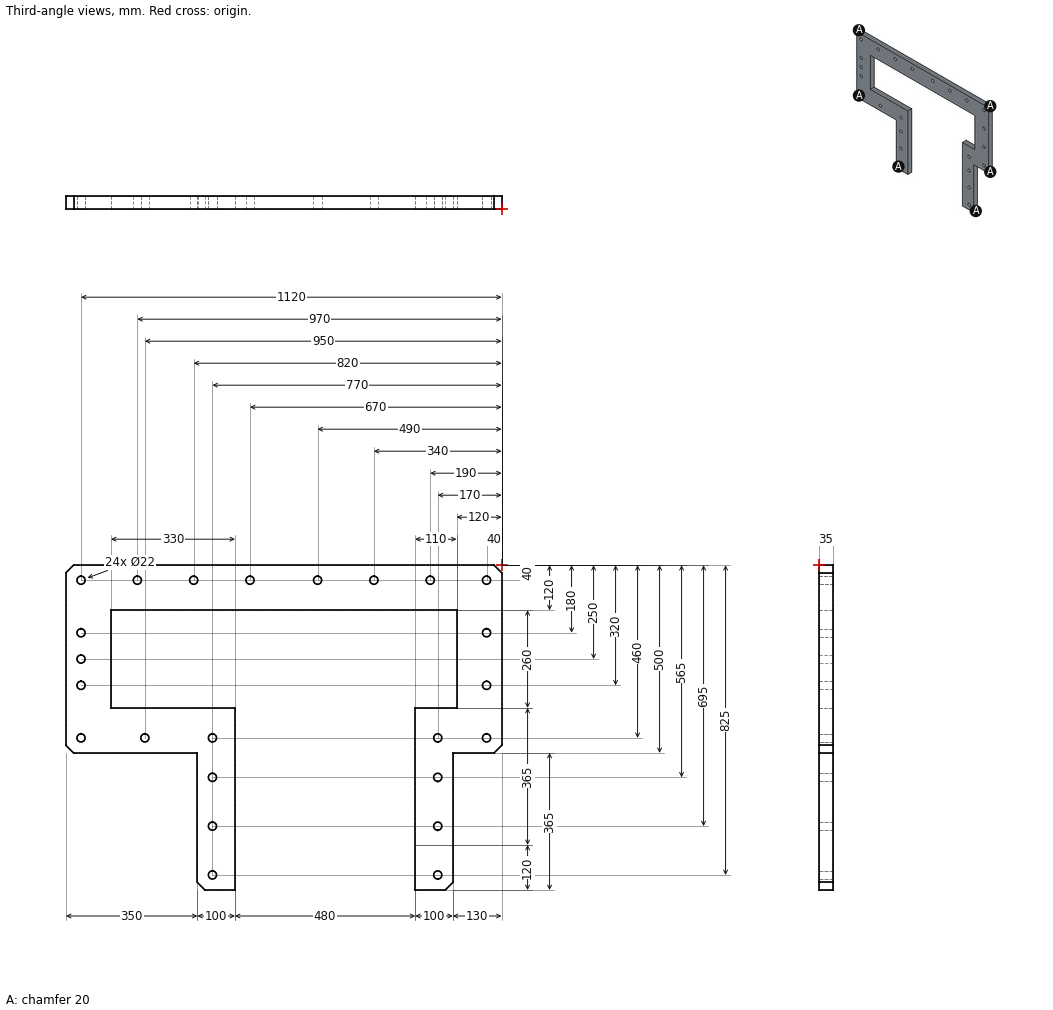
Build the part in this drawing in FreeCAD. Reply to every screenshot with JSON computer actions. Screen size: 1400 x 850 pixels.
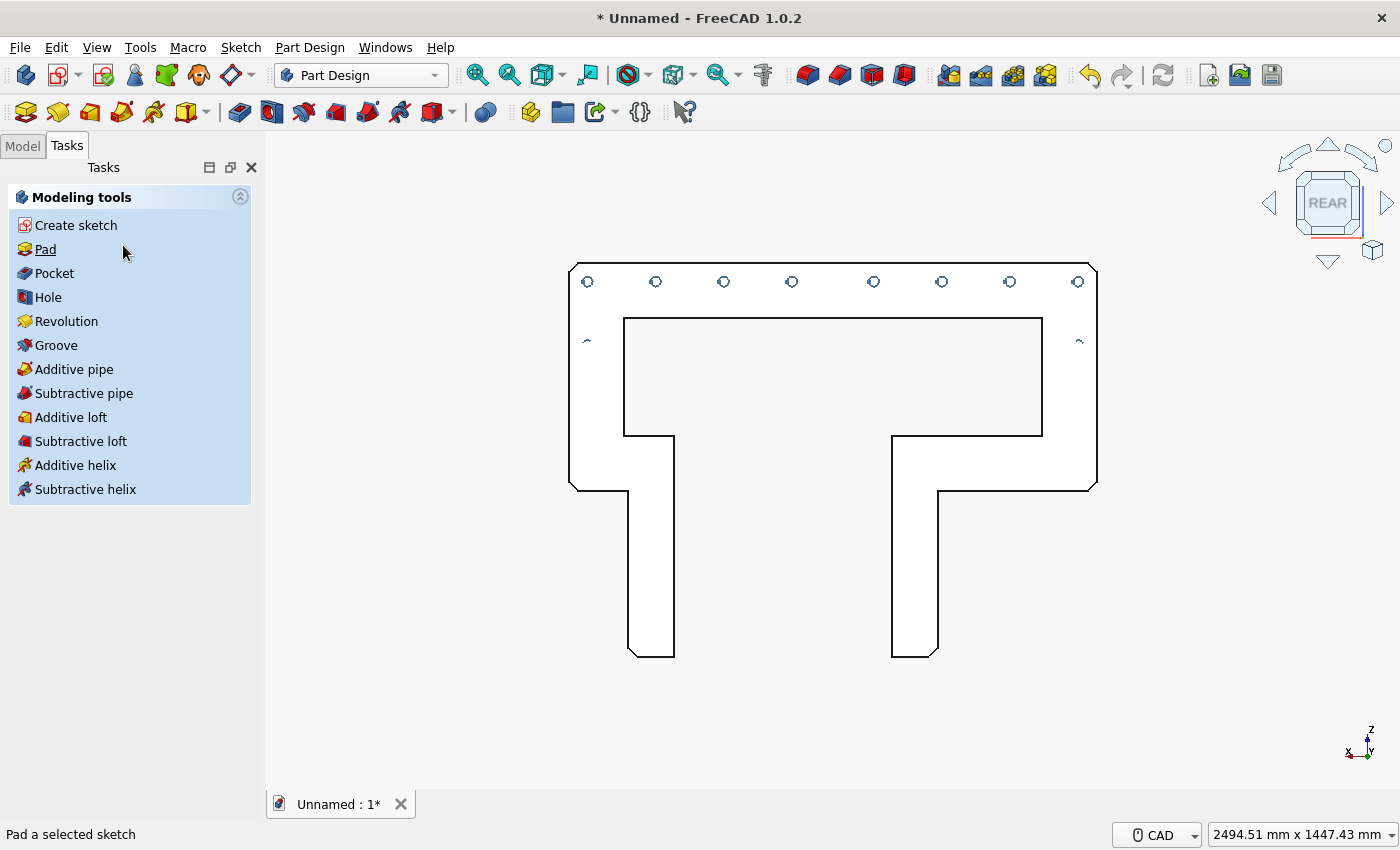
{"action": "left_click", "coordinate": [240, 112]}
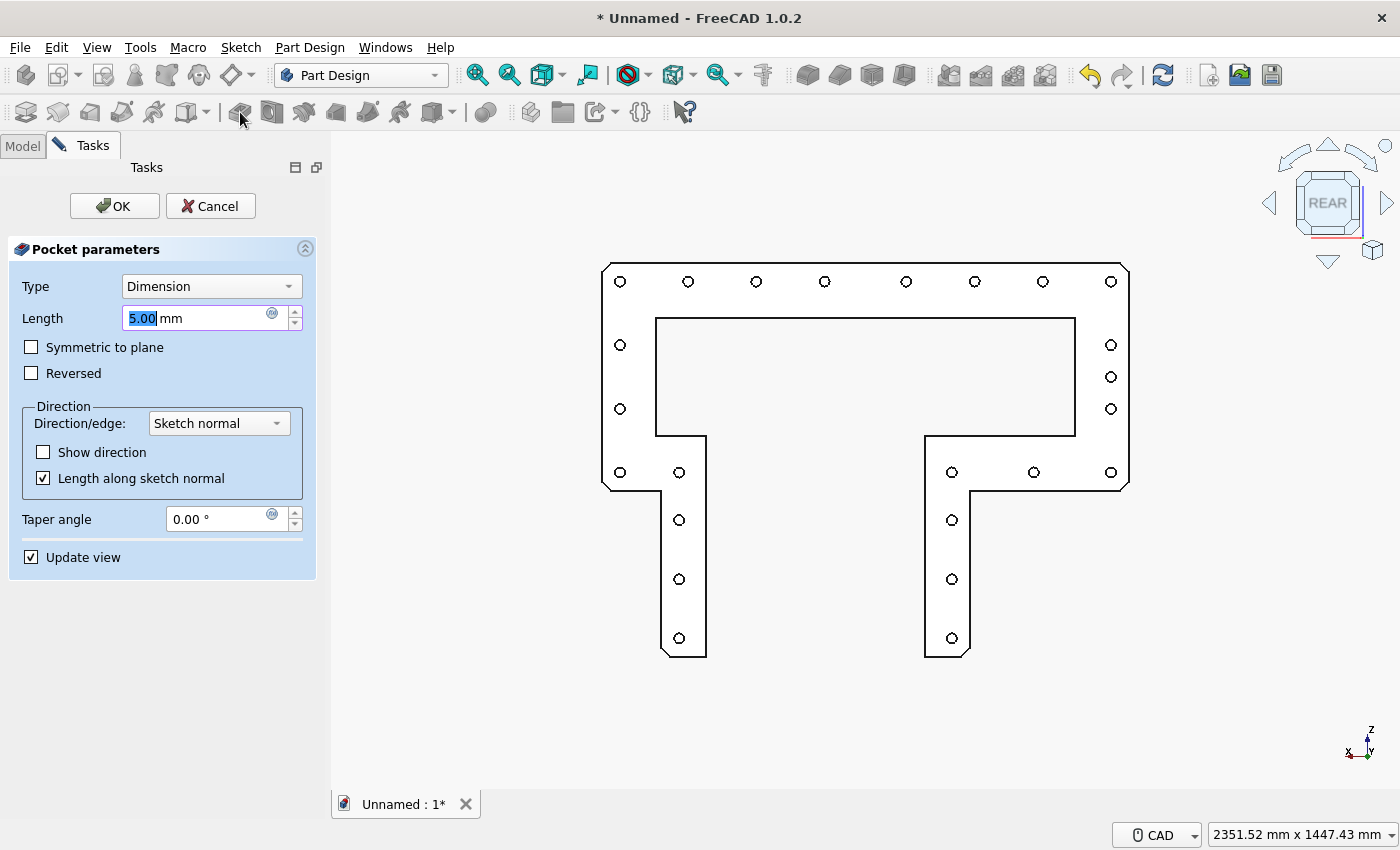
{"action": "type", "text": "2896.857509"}
{"action": "key", "text": "Tab"}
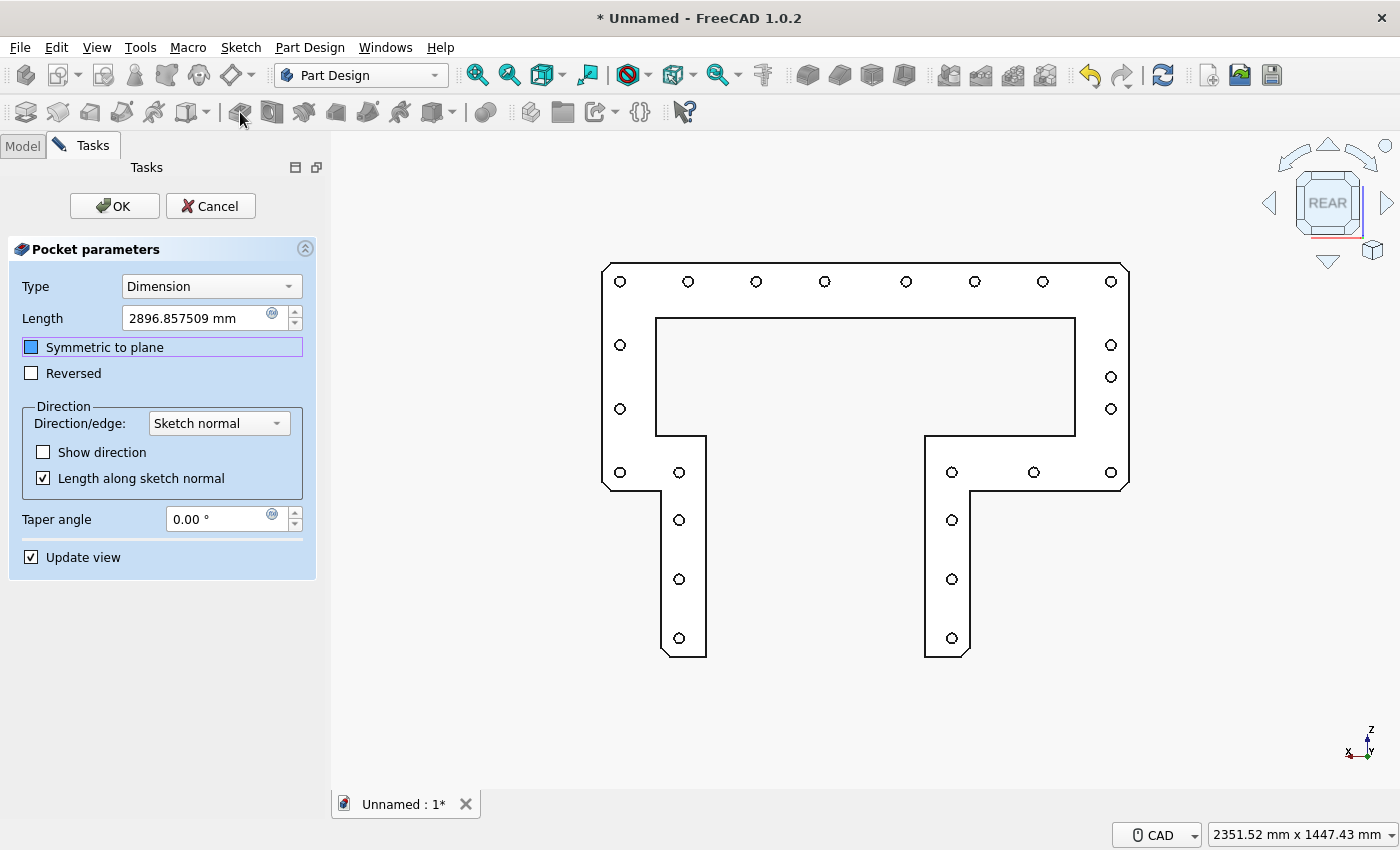
{"action": "left_click", "coordinate": [30, 347]}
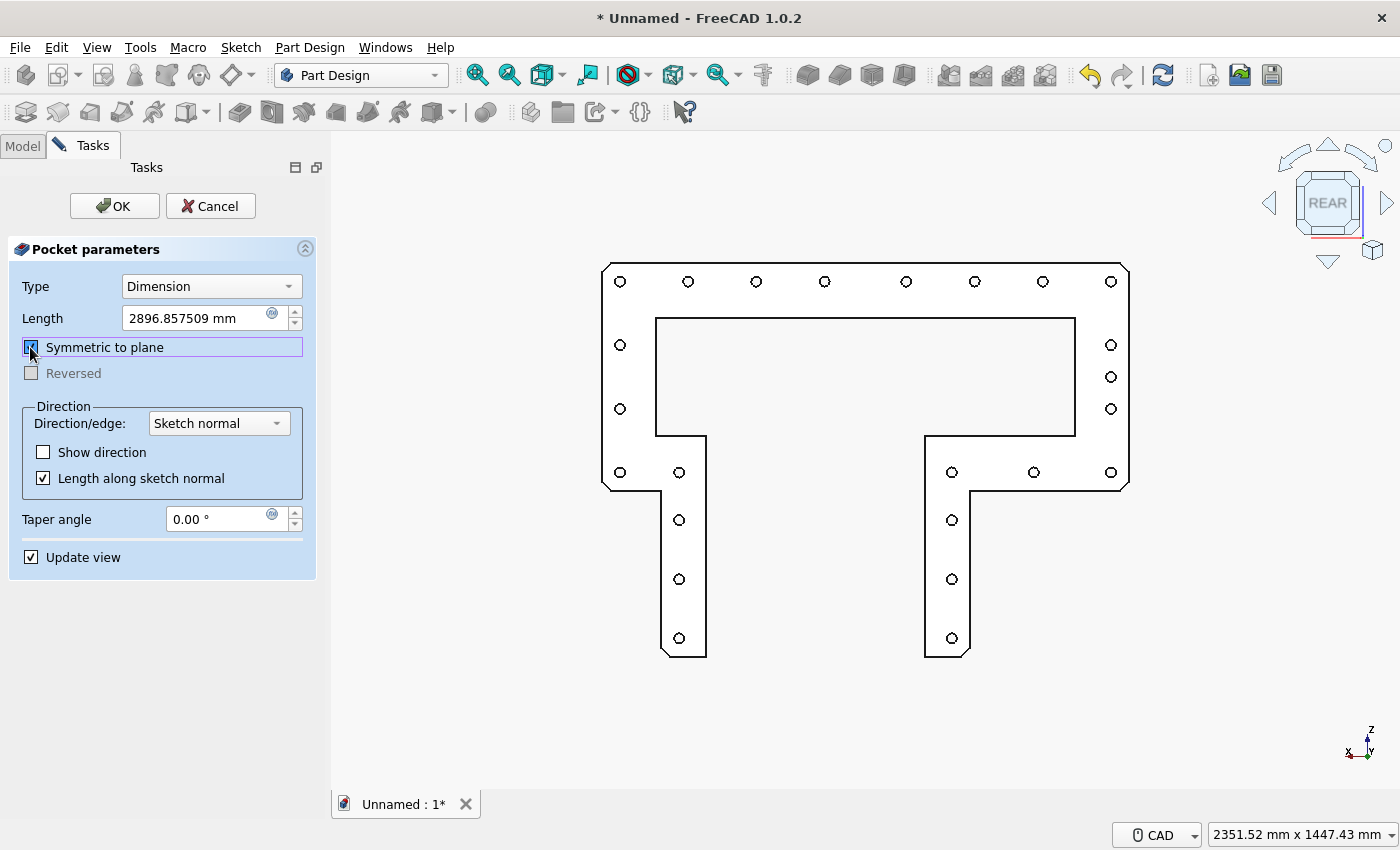
{"action": "left_click", "coordinate": [115, 206]}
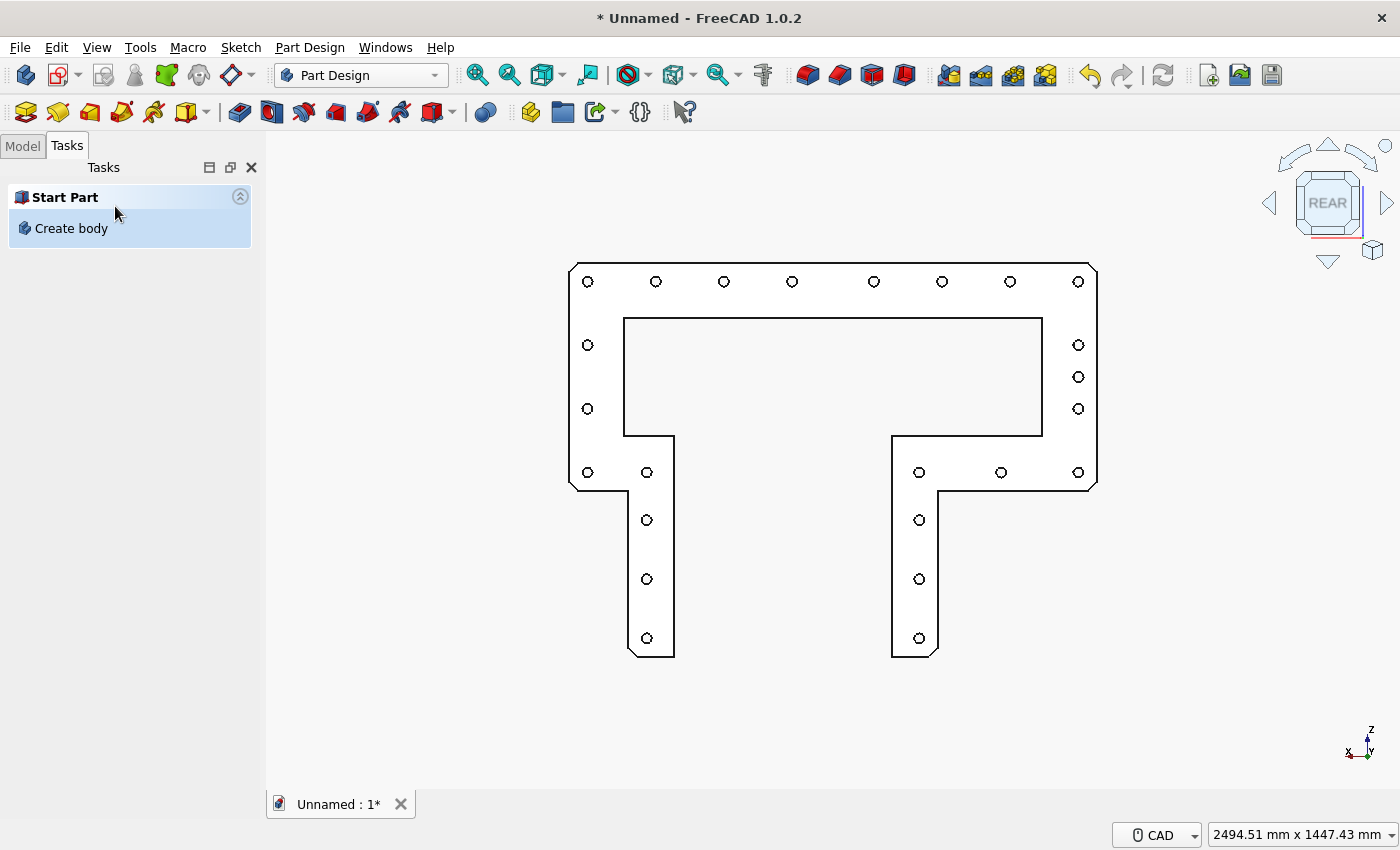
{"action": "key", "text": "0"}